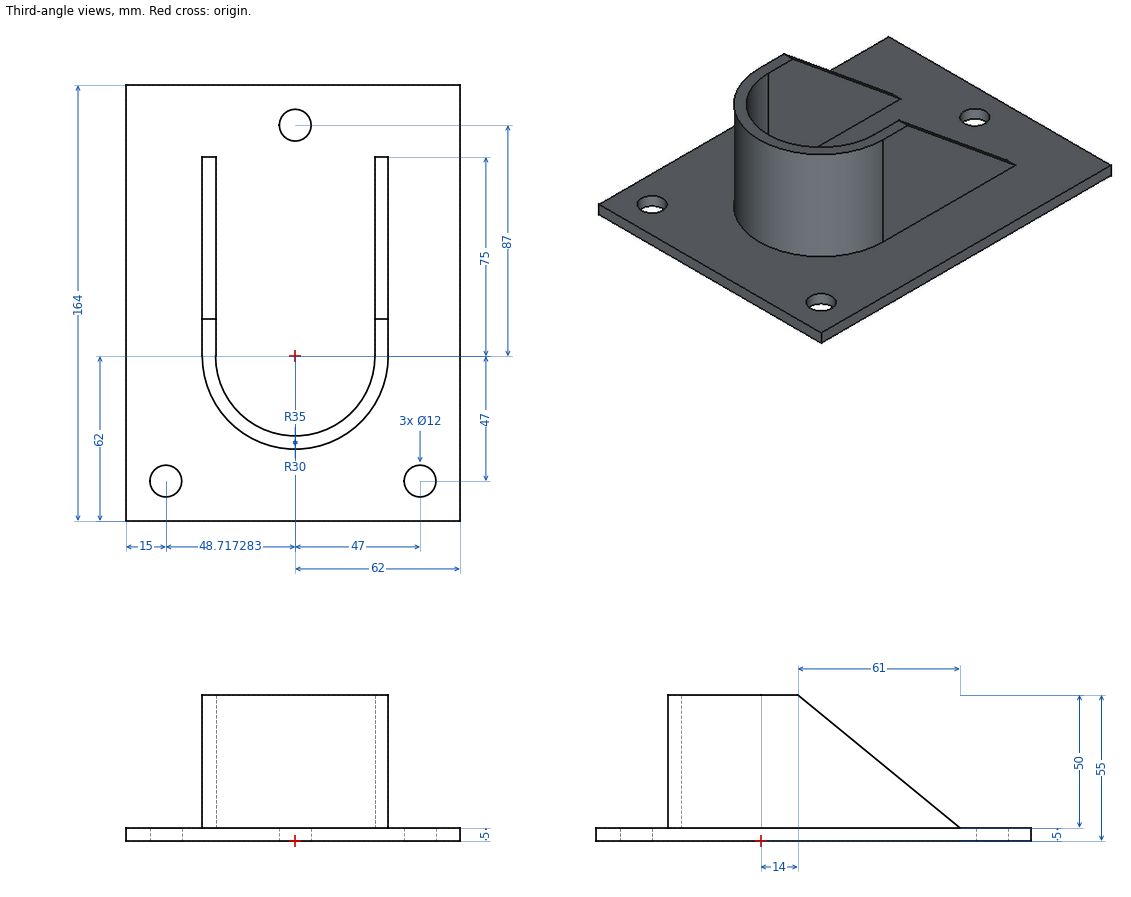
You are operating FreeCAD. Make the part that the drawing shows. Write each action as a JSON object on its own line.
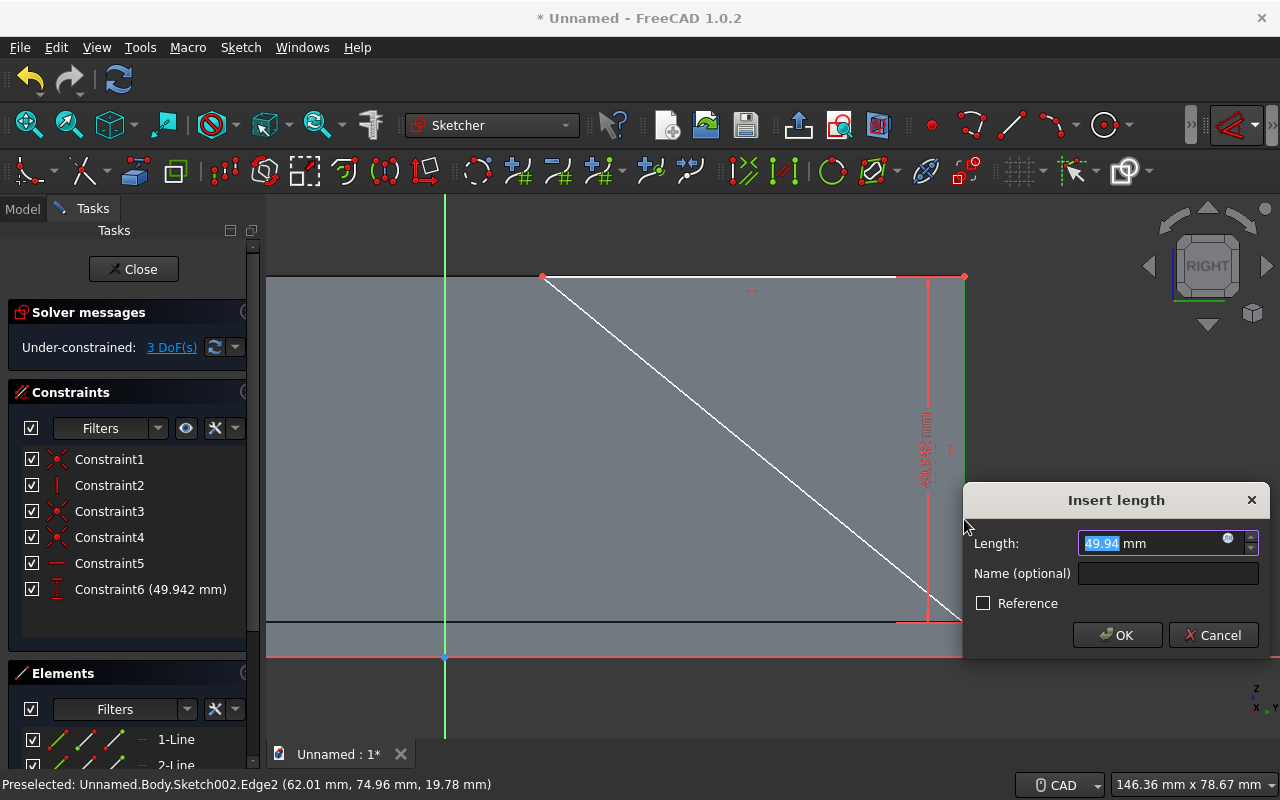
{"action": "type", "text": "50"}
{"action": "key", "text": "Return"}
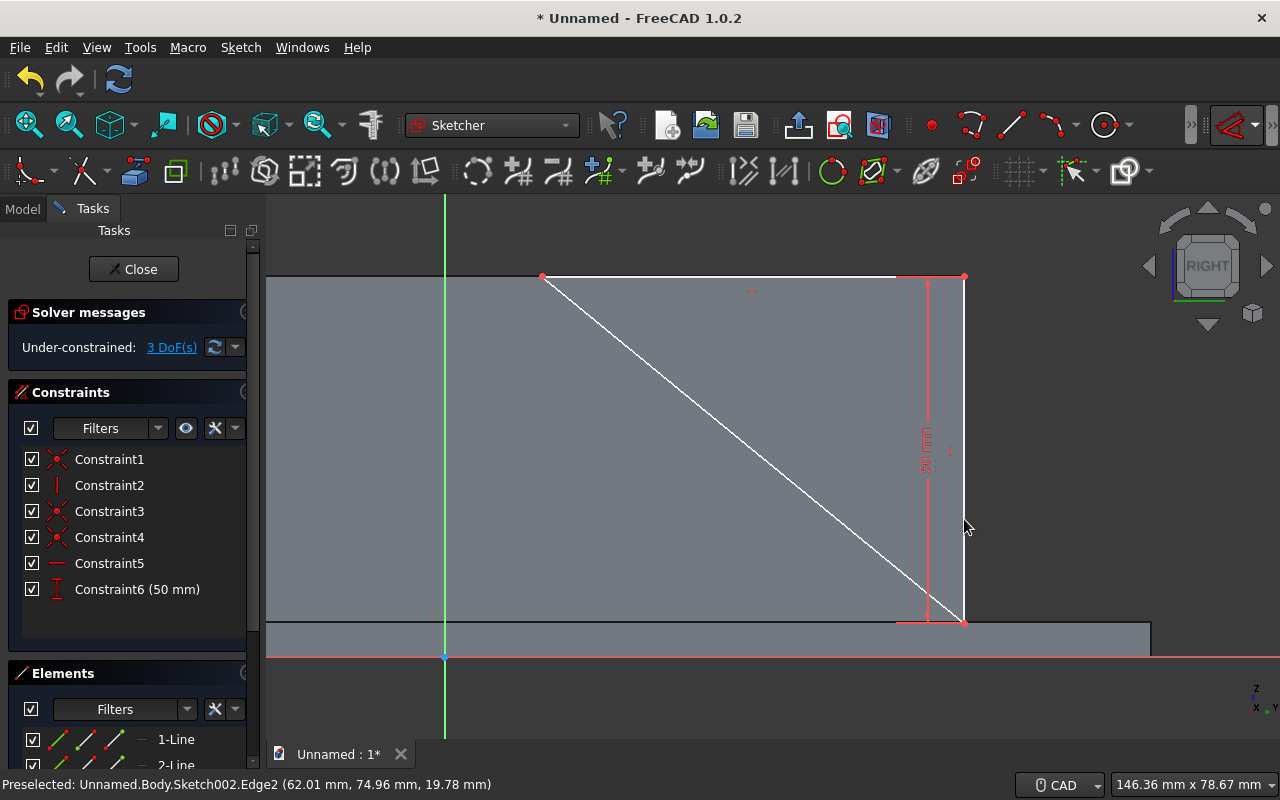
{"action": "left_click", "coordinate": [837, 277]}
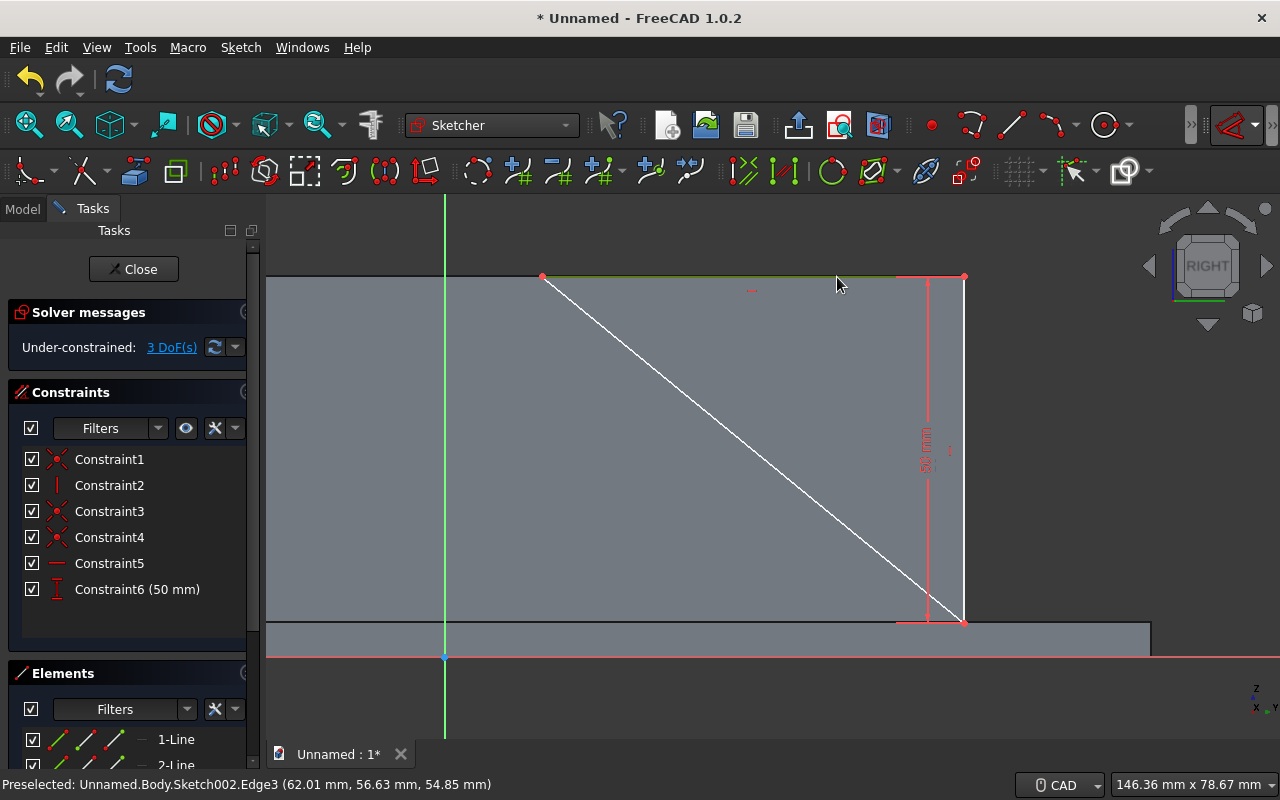
{"action": "left_click", "coordinate": [1258, 126]}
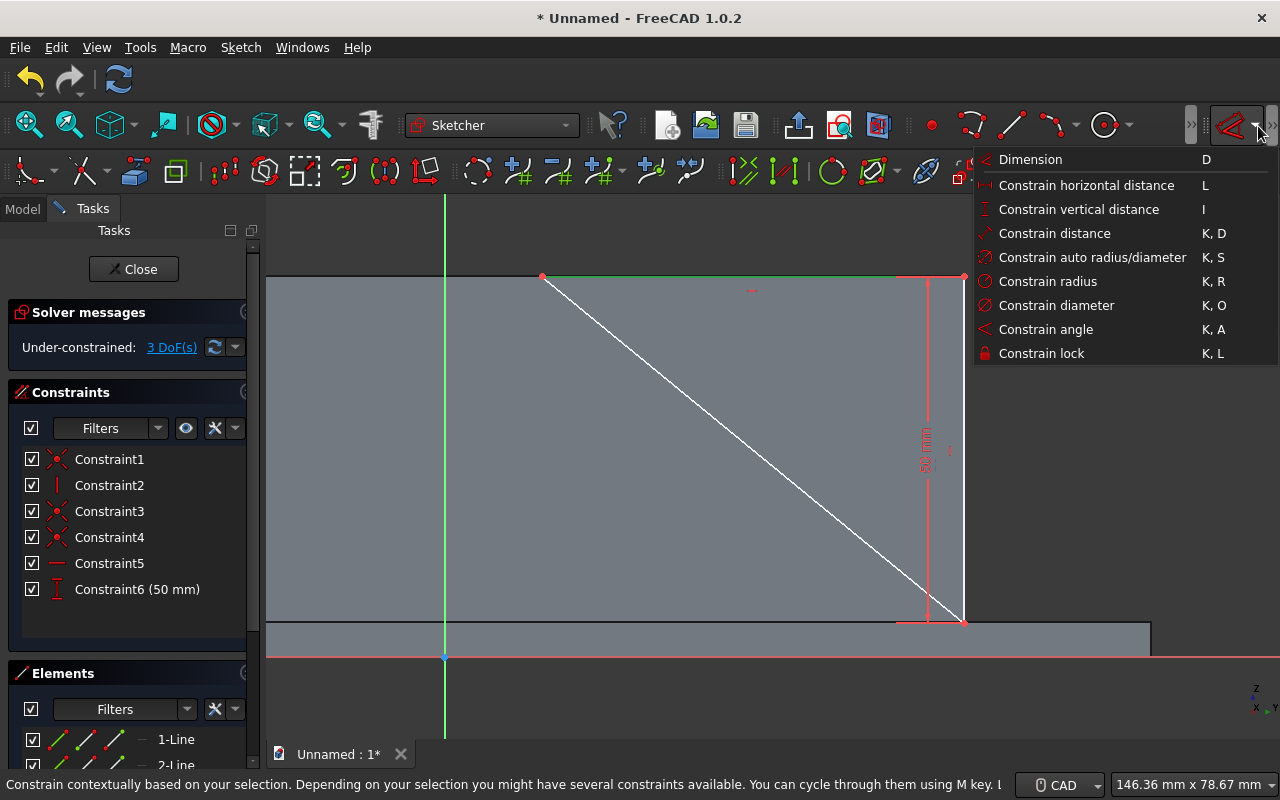
{"action": "left_click", "coordinate": [1126, 185]}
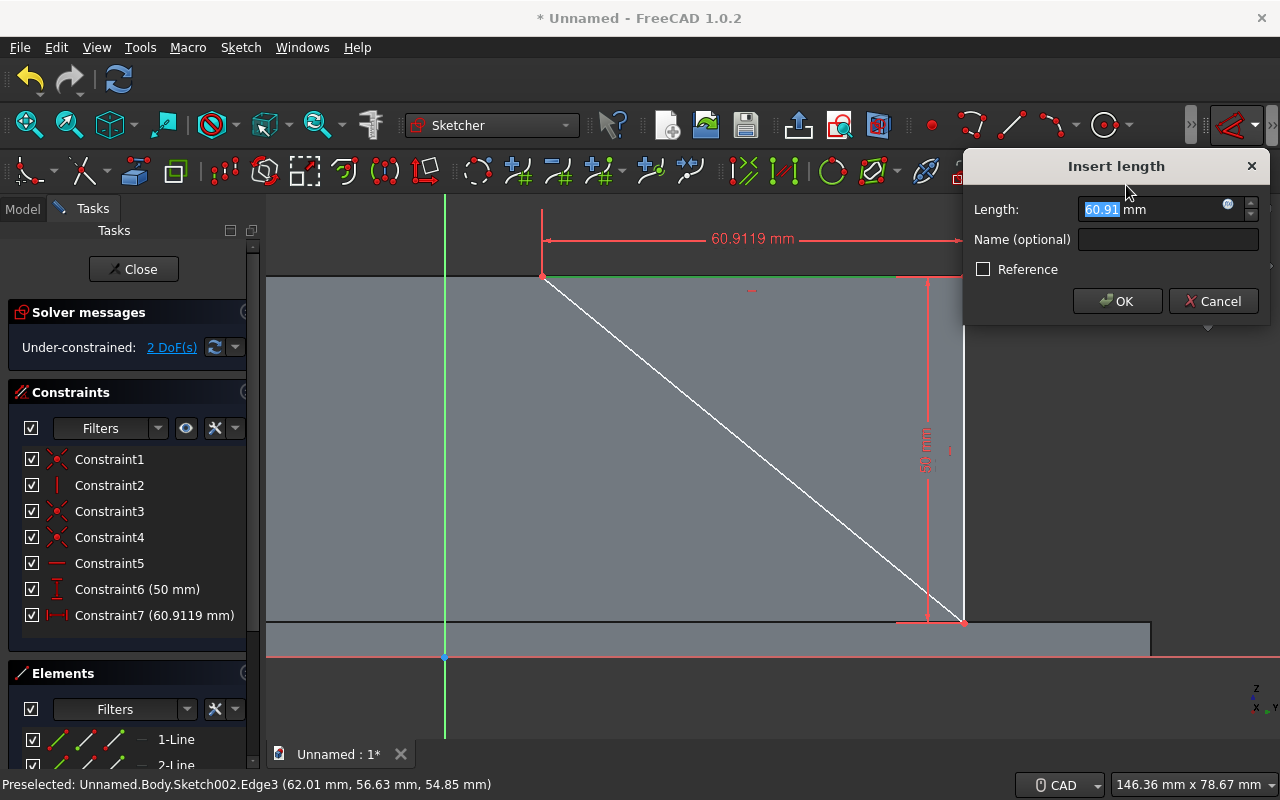
{"action": "type", "text": "61"}
{"action": "key", "text": "Return"}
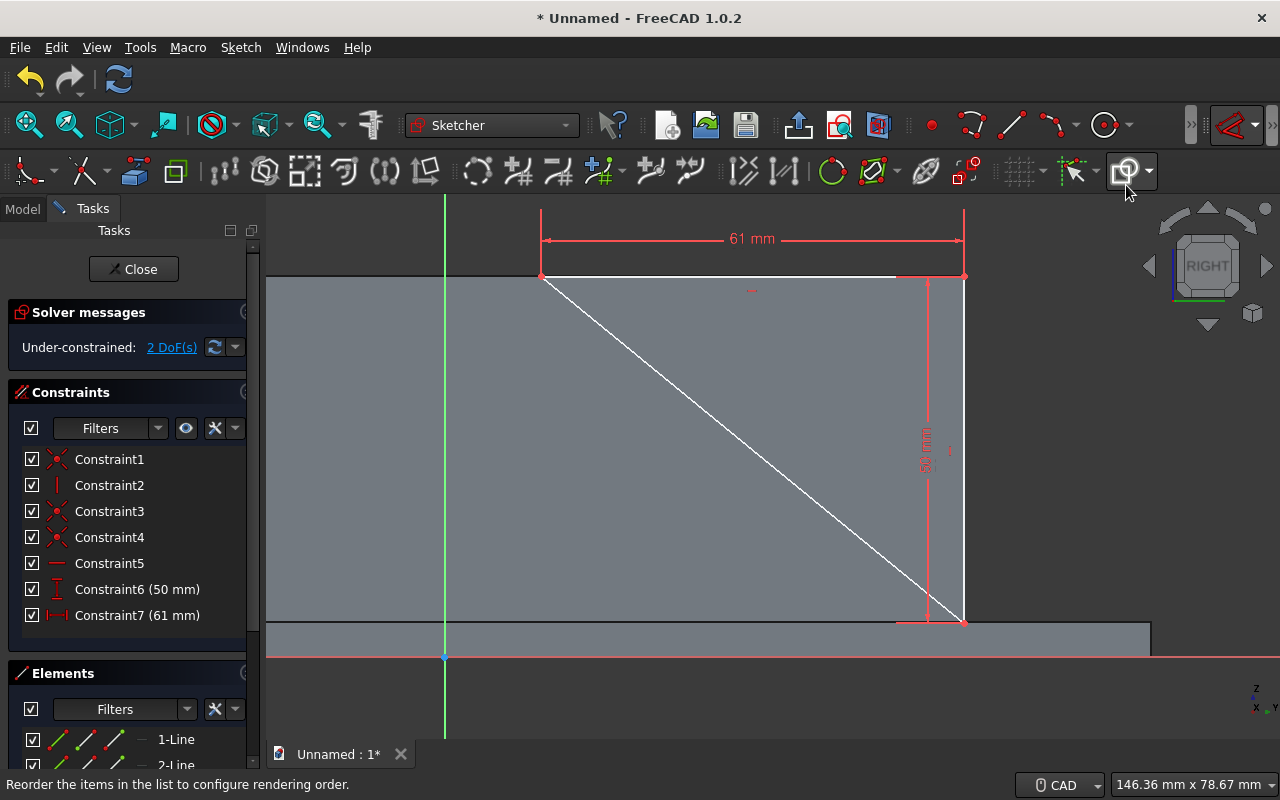
{"action": "left_click", "coordinate": [964, 623]}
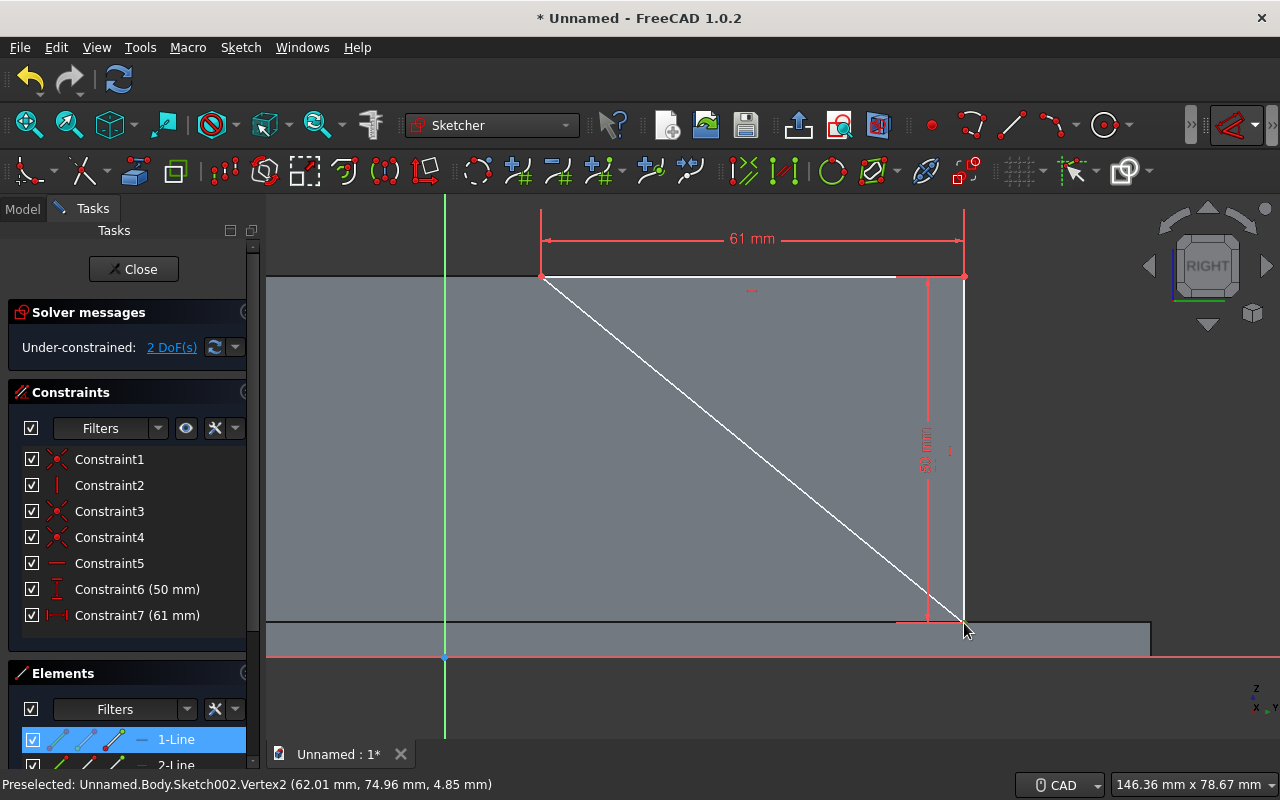
{"action": "key", "text": "i"}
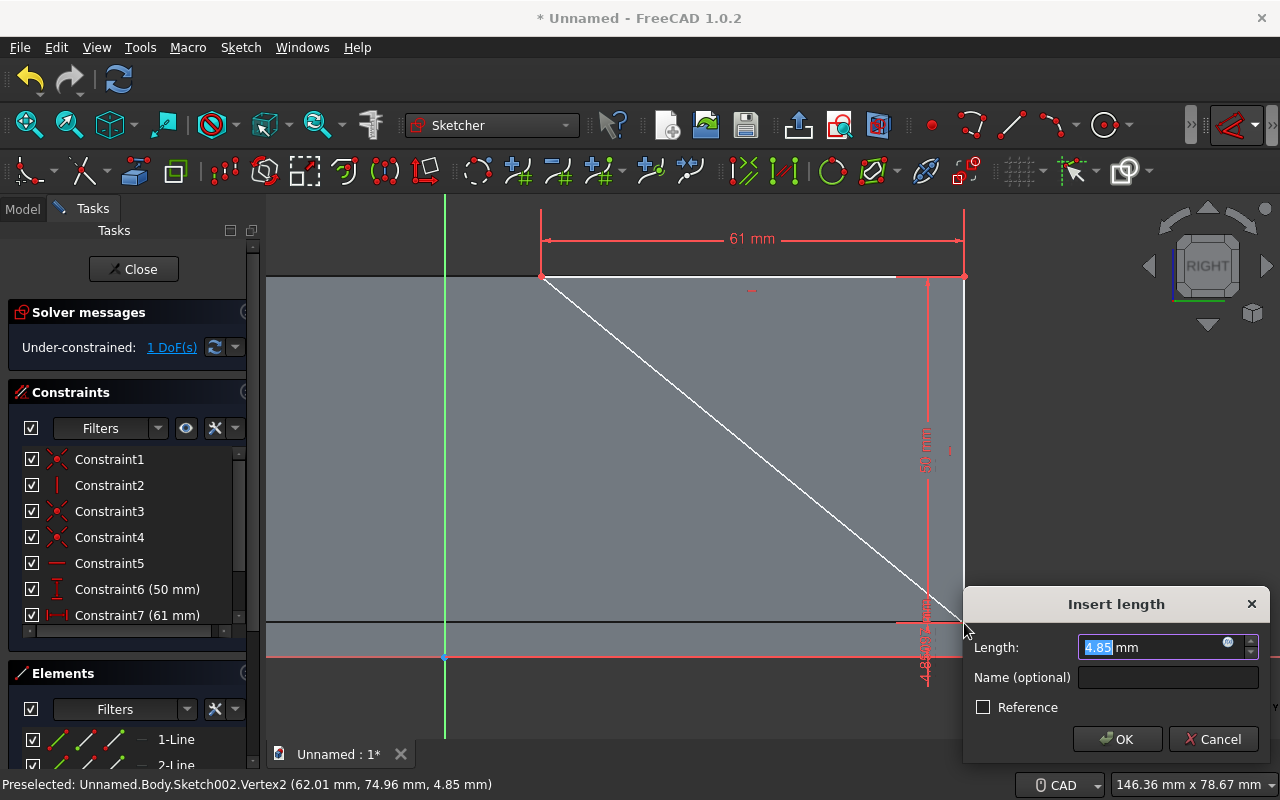
{"action": "type", "text": "5"}
{"action": "key", "text": "Return"}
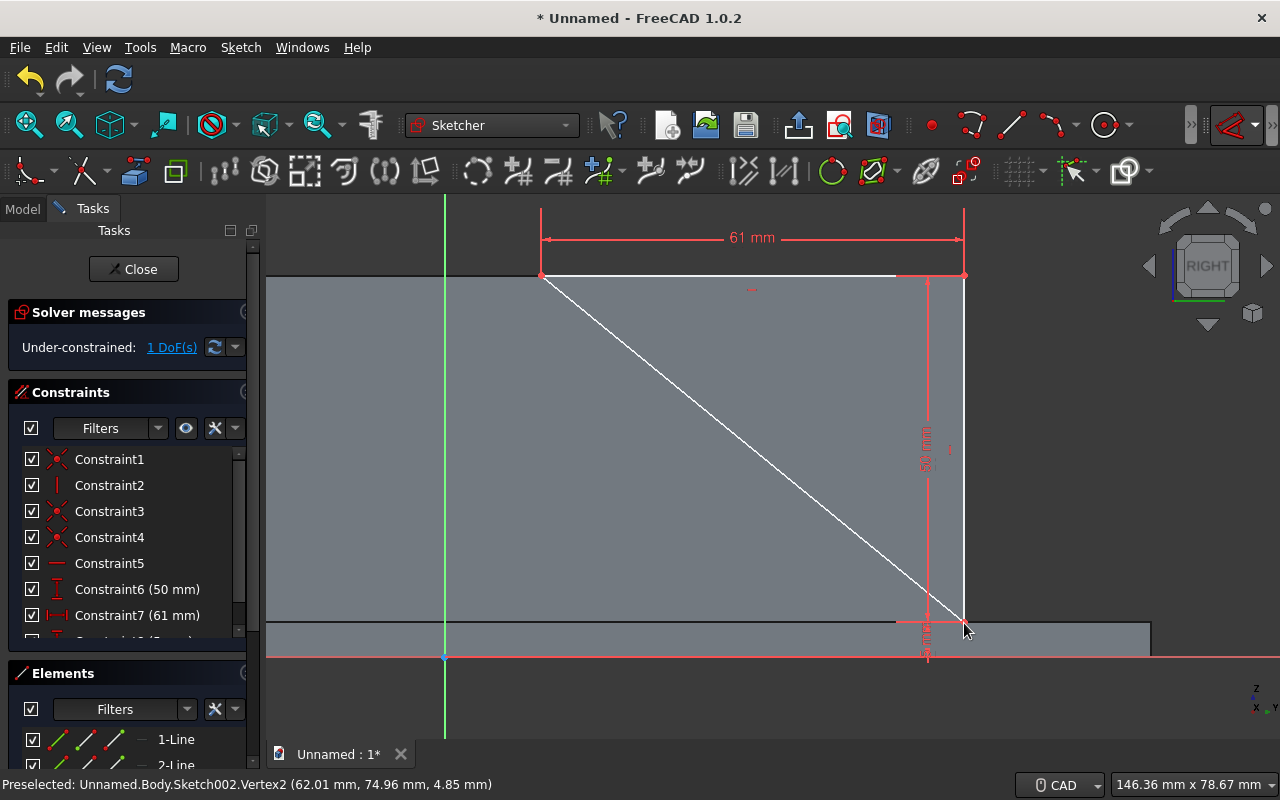
{"action": "left_click", "coordinate": [541, 276]}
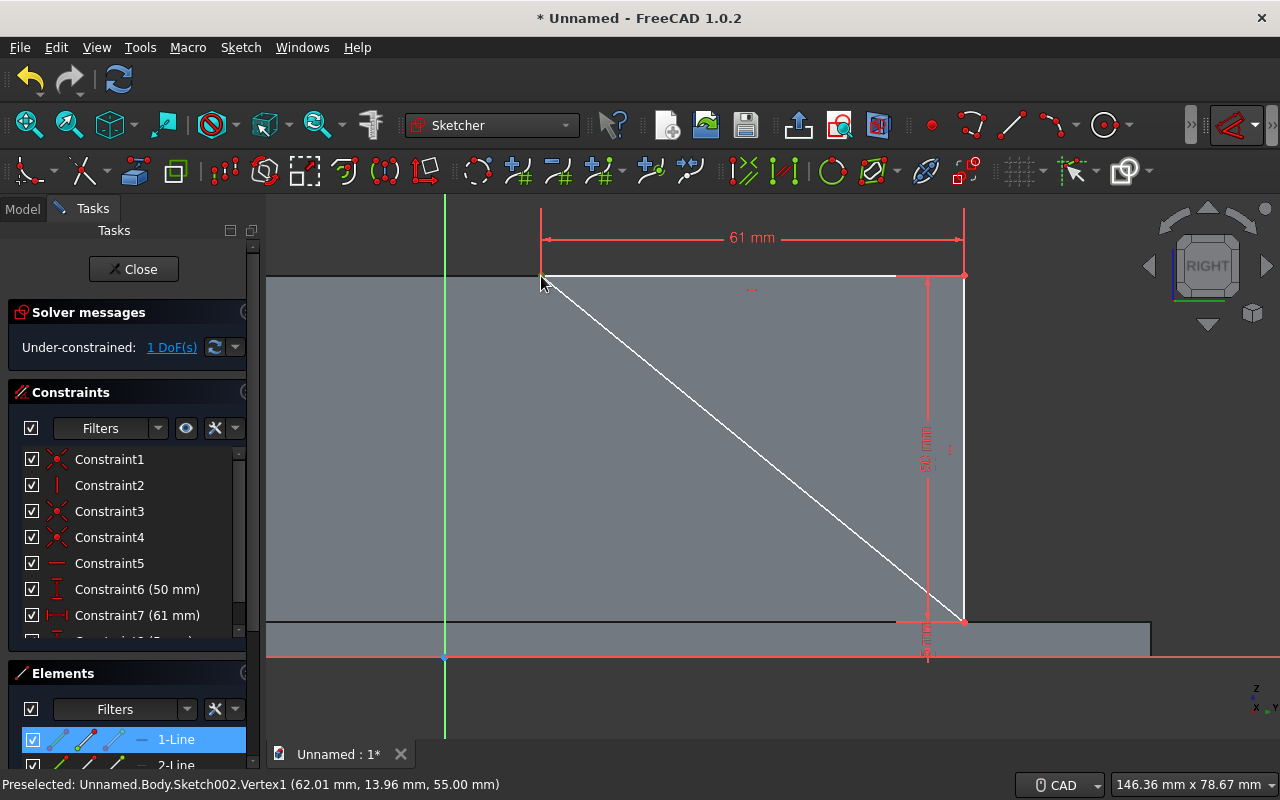
{"action": "left_click", "coordinate": [1258, 126]}